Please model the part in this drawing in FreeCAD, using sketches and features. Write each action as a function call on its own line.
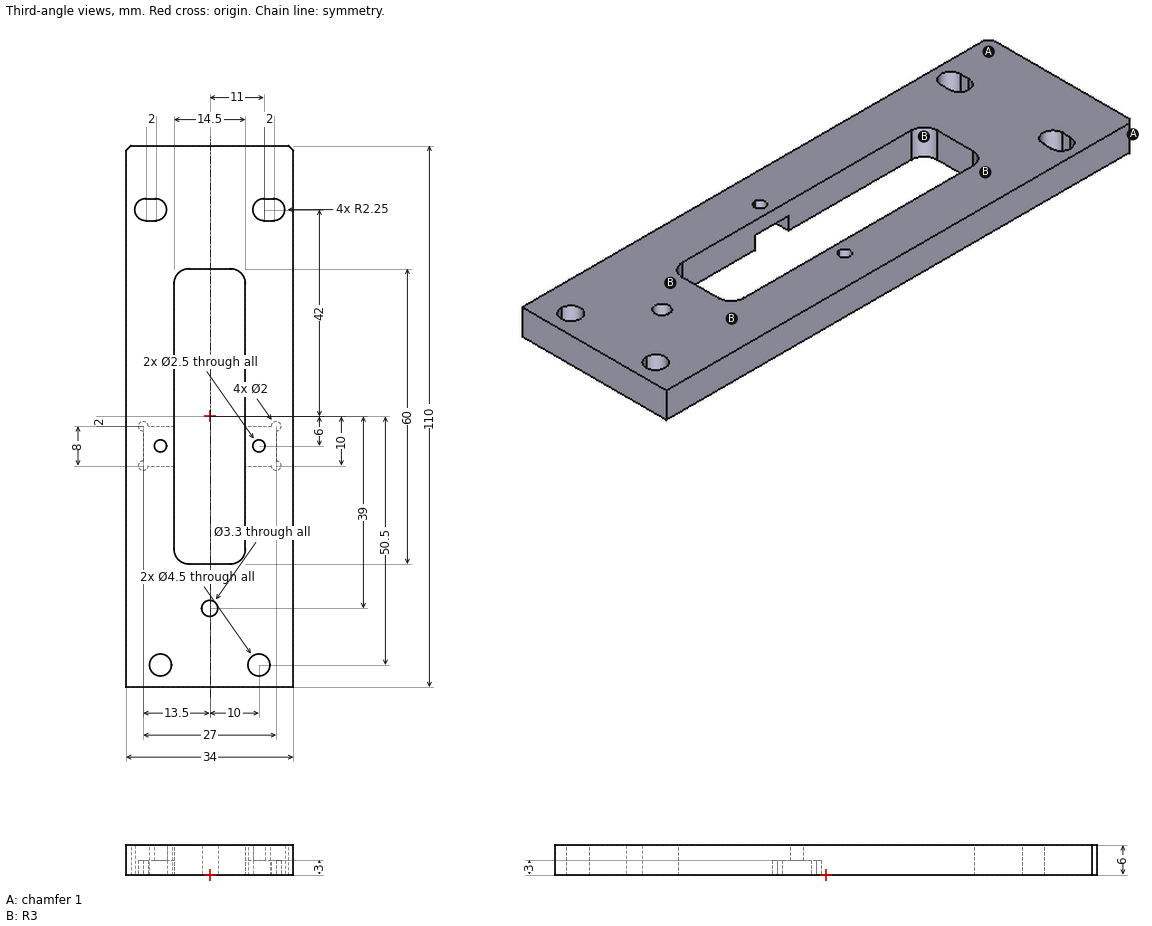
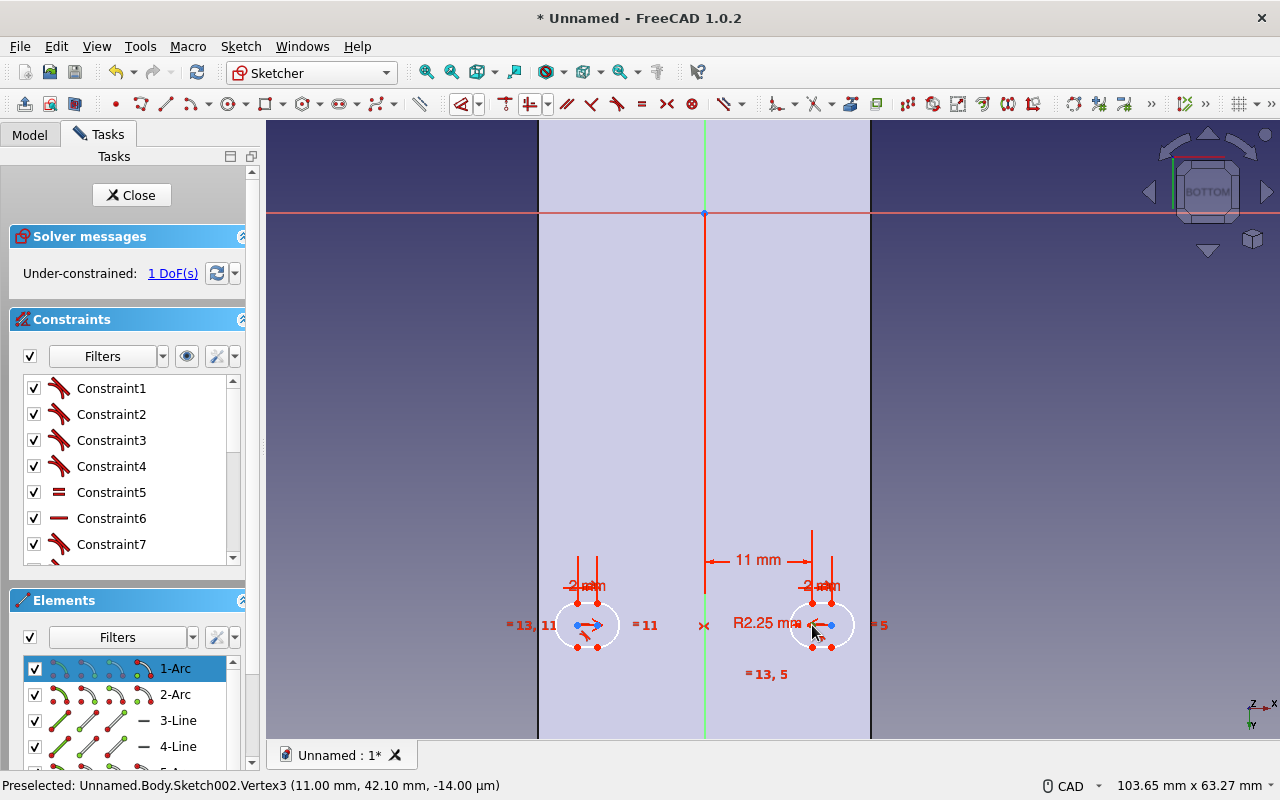
key(i)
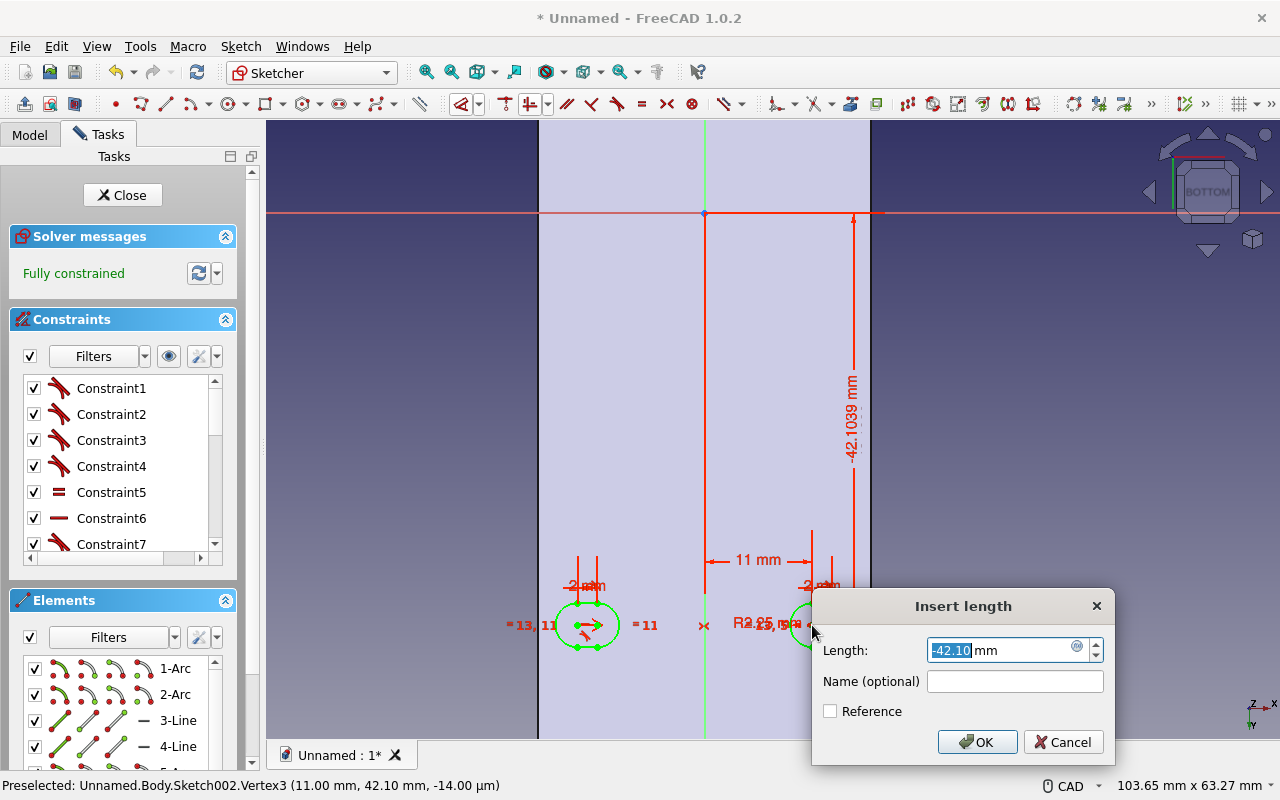
text(-42)
key(Return)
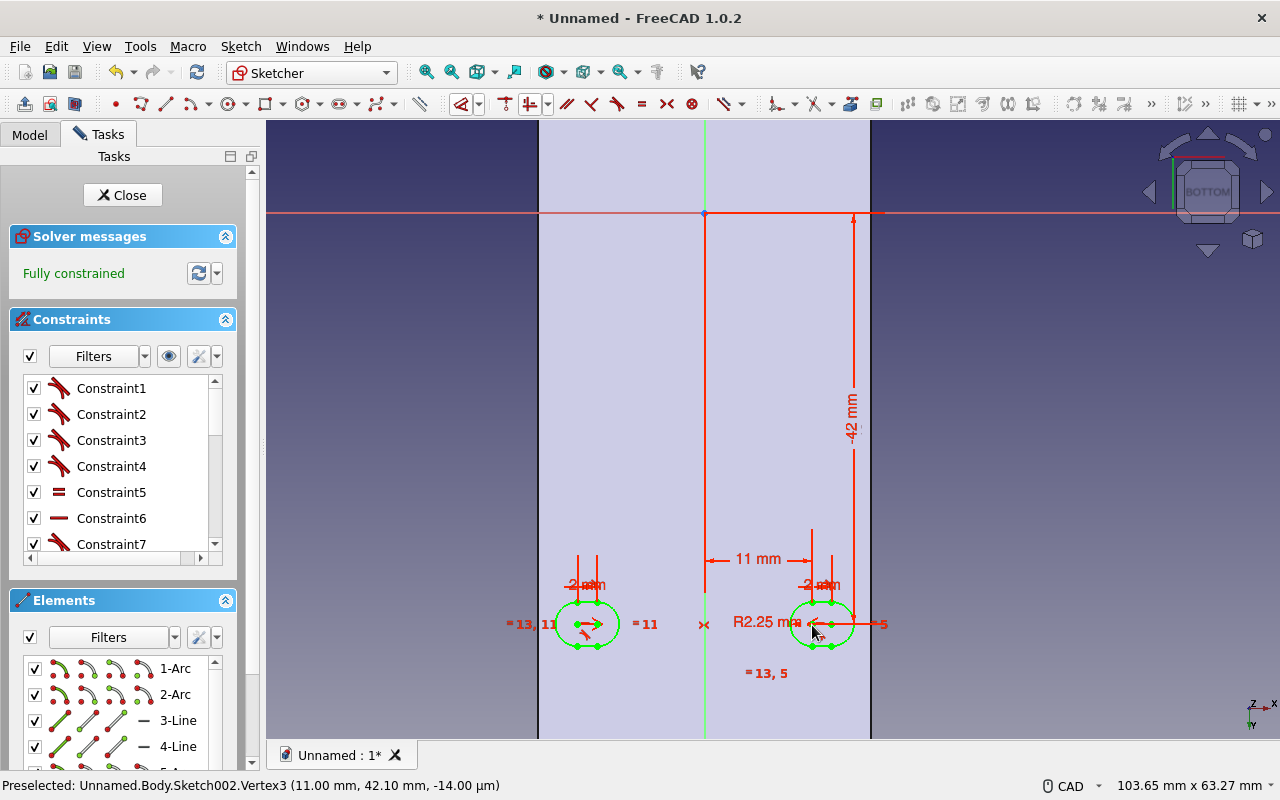
click(123, 195)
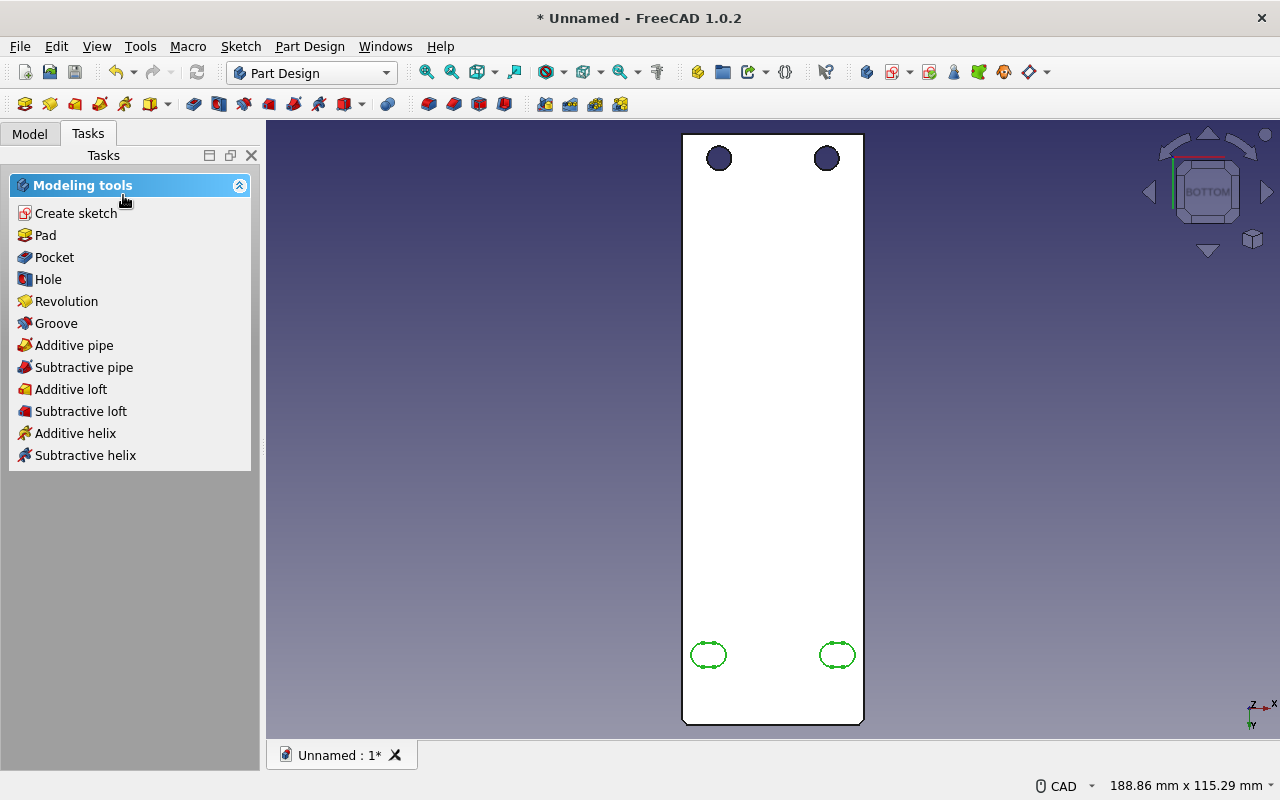
click(194, 104)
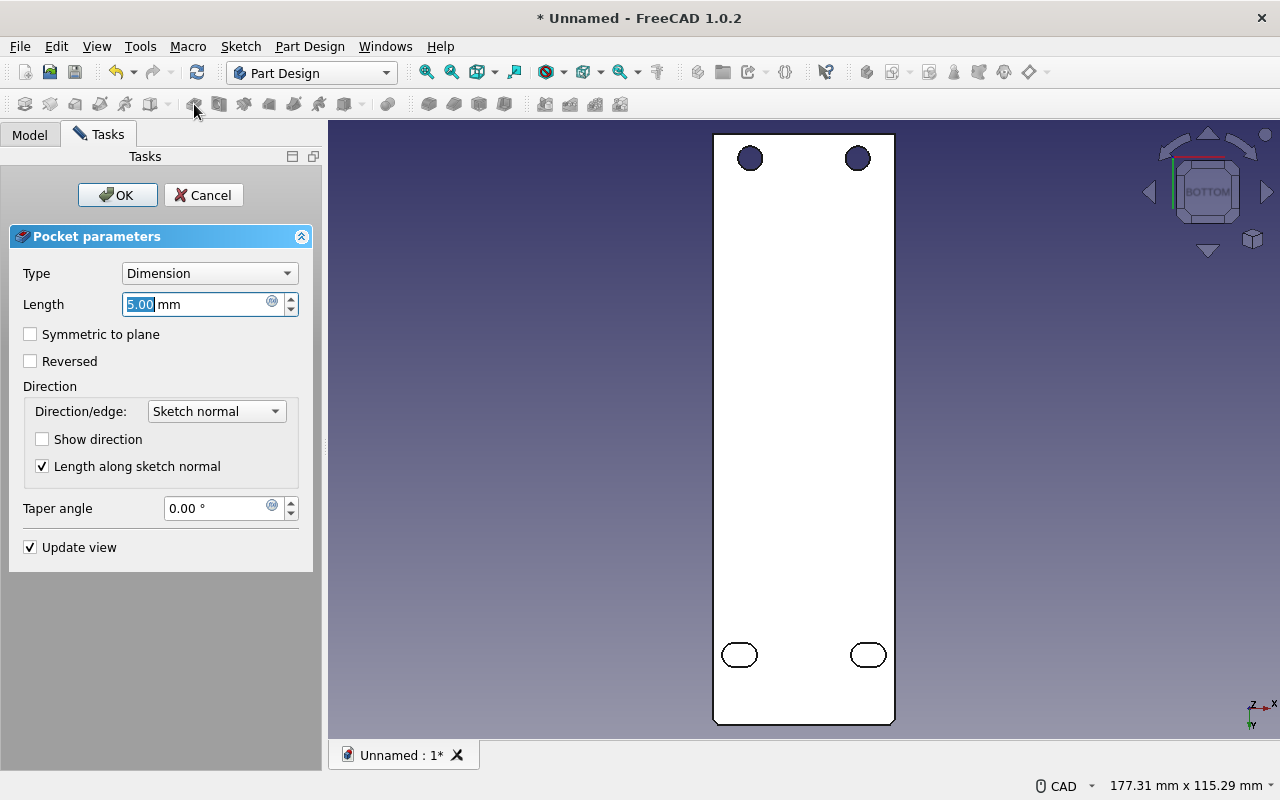
click(210, 274)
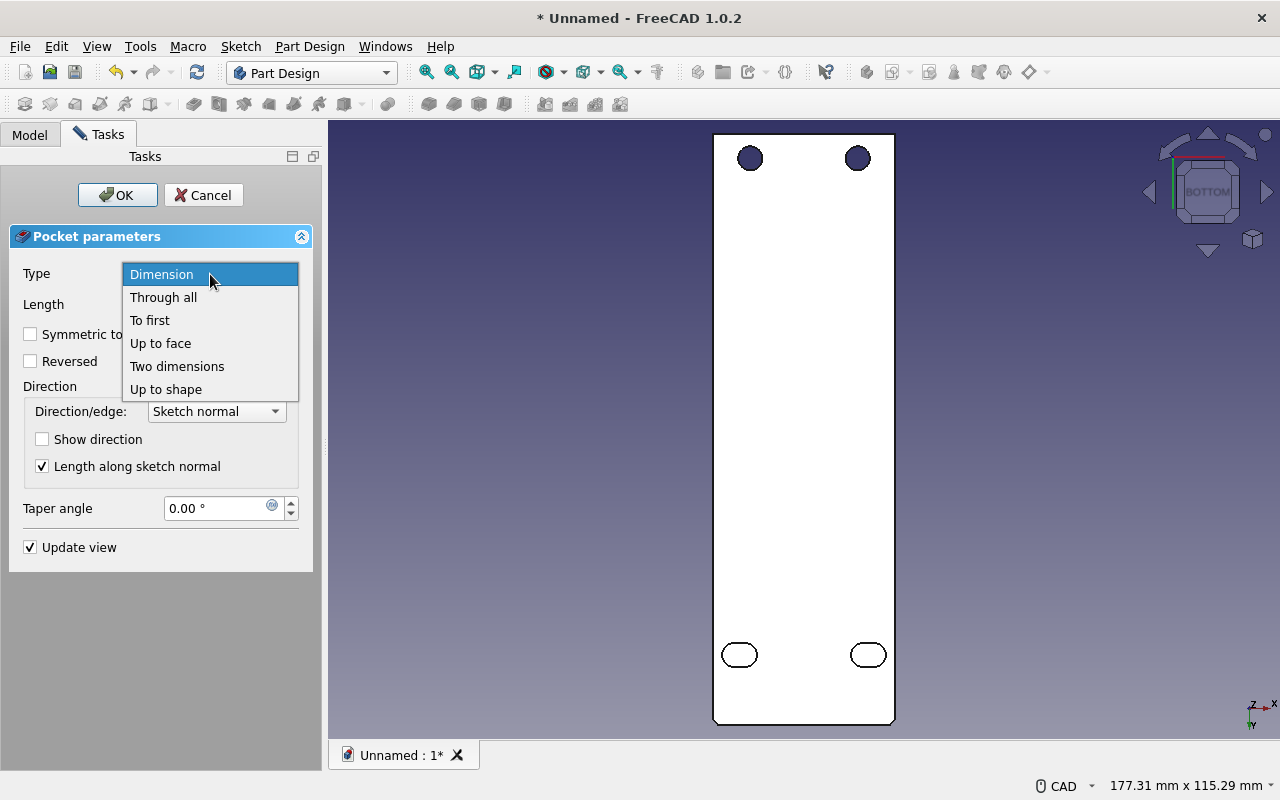
click(208, 298)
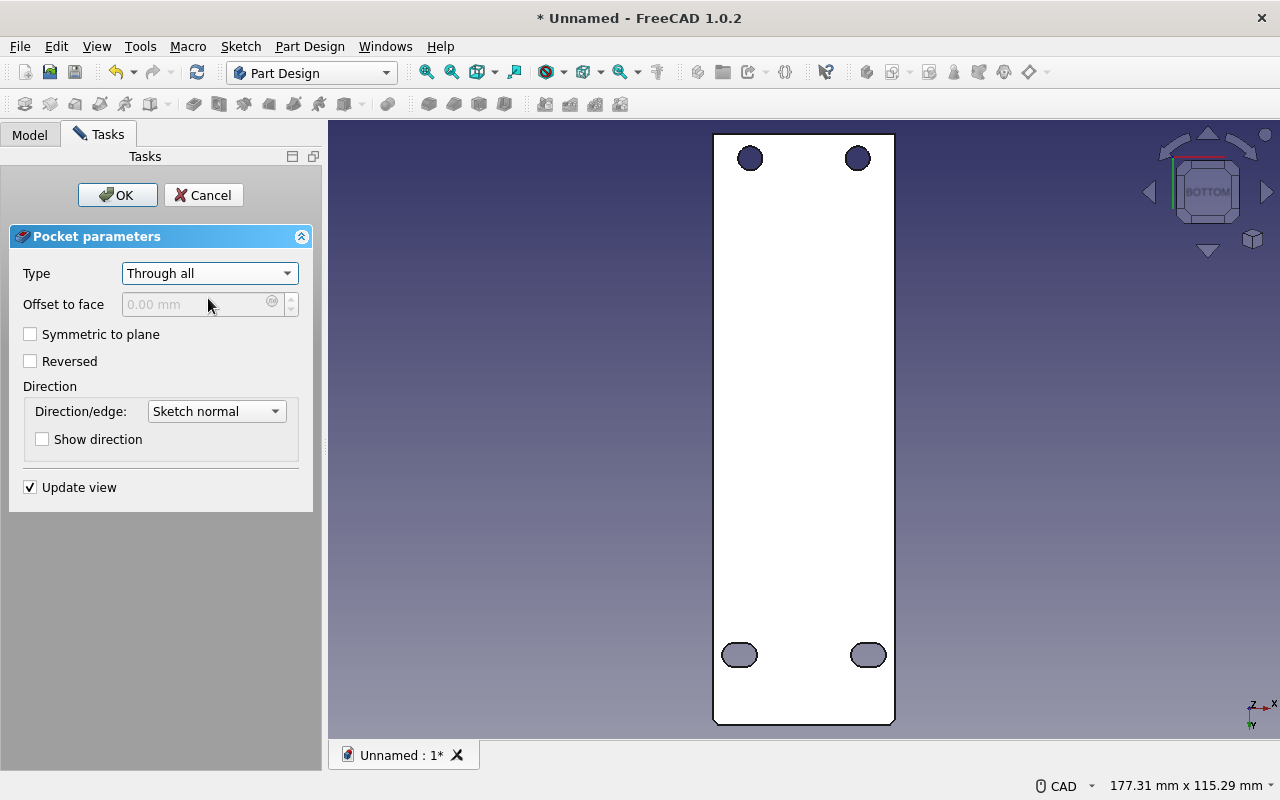
click(118, 195)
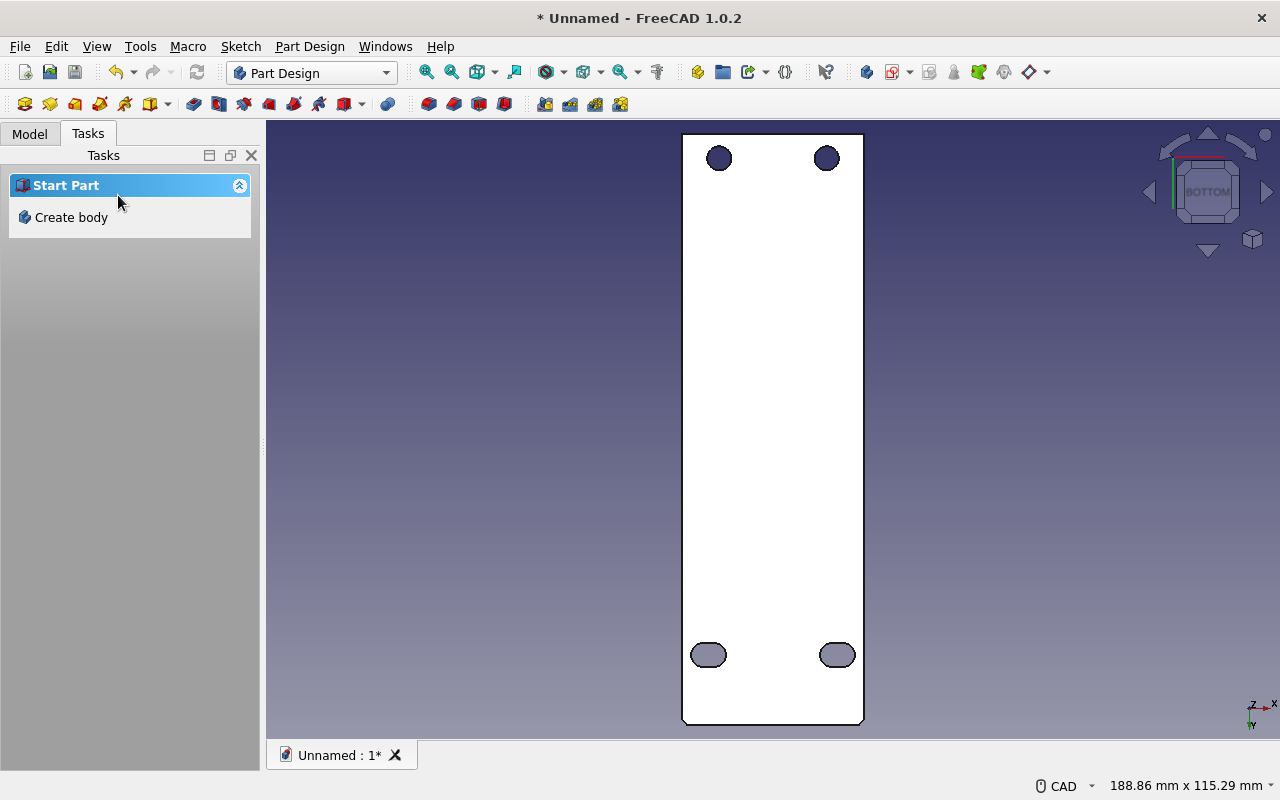
click(773, 513)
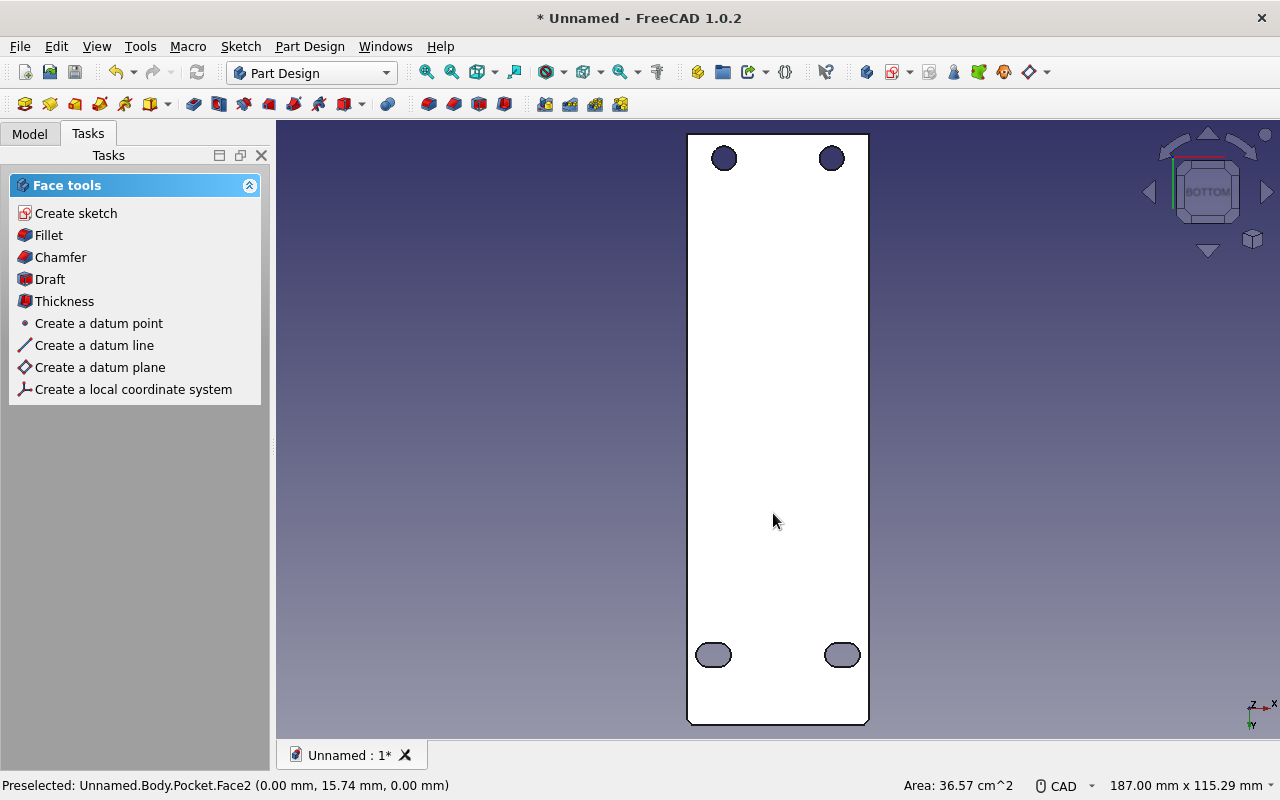
click(892, 72)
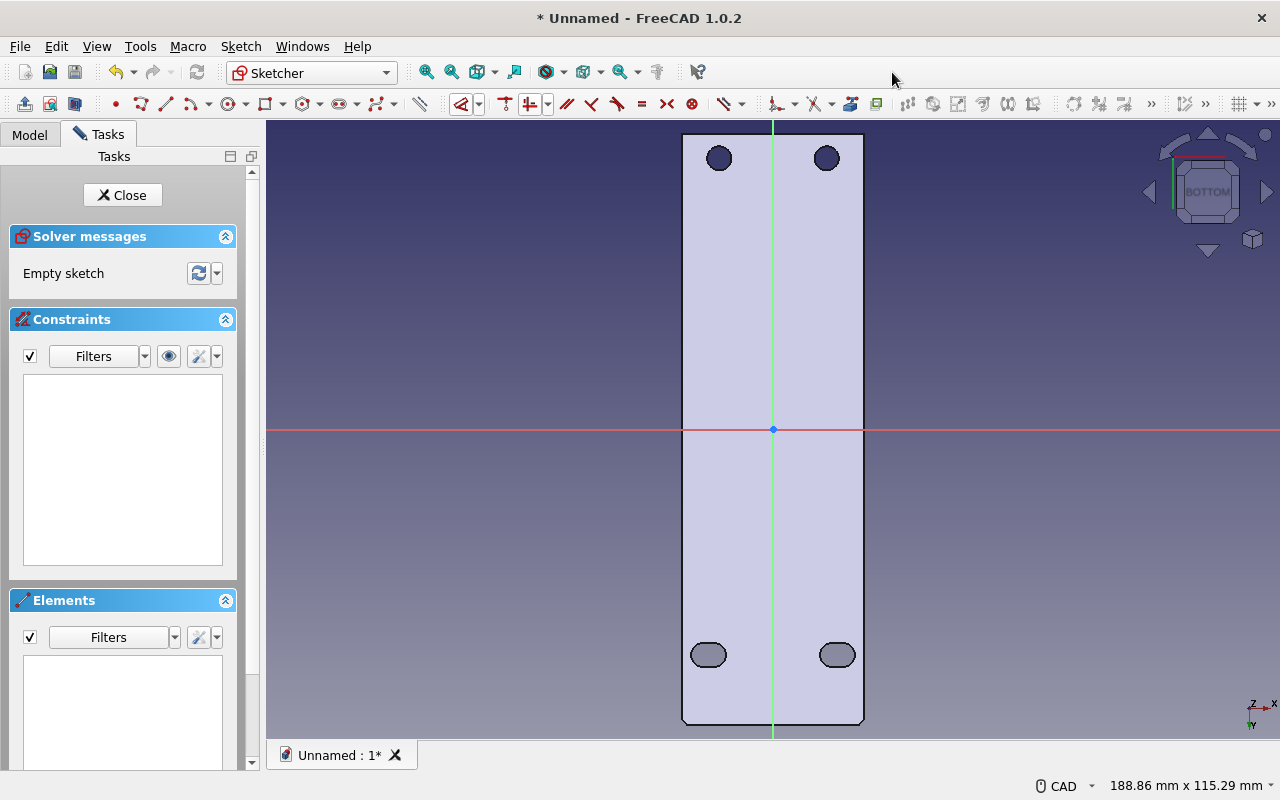
key(g)
key(v)